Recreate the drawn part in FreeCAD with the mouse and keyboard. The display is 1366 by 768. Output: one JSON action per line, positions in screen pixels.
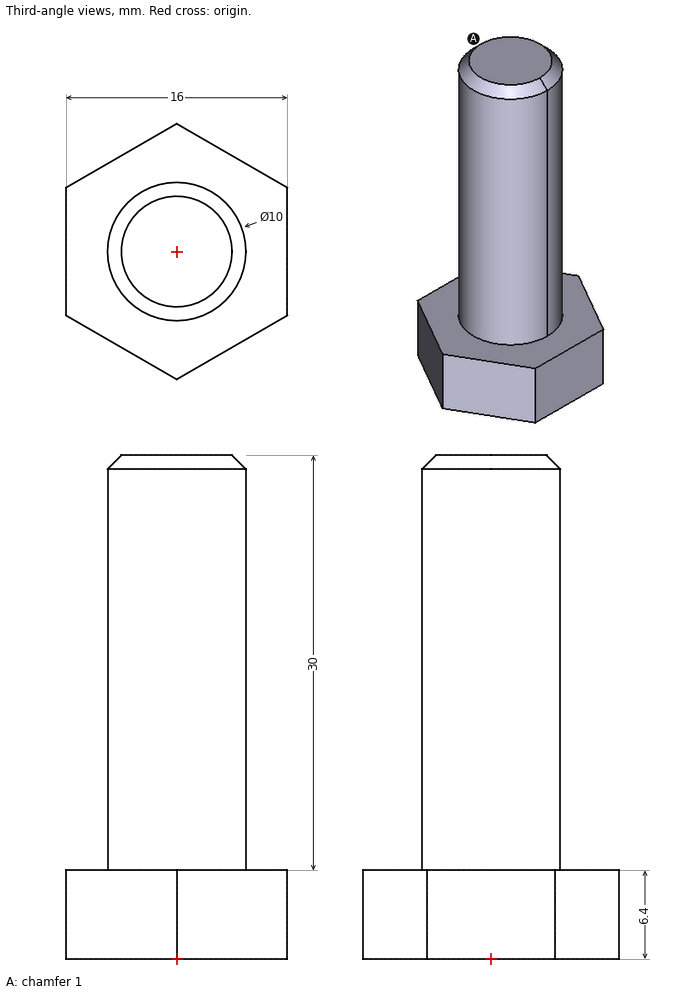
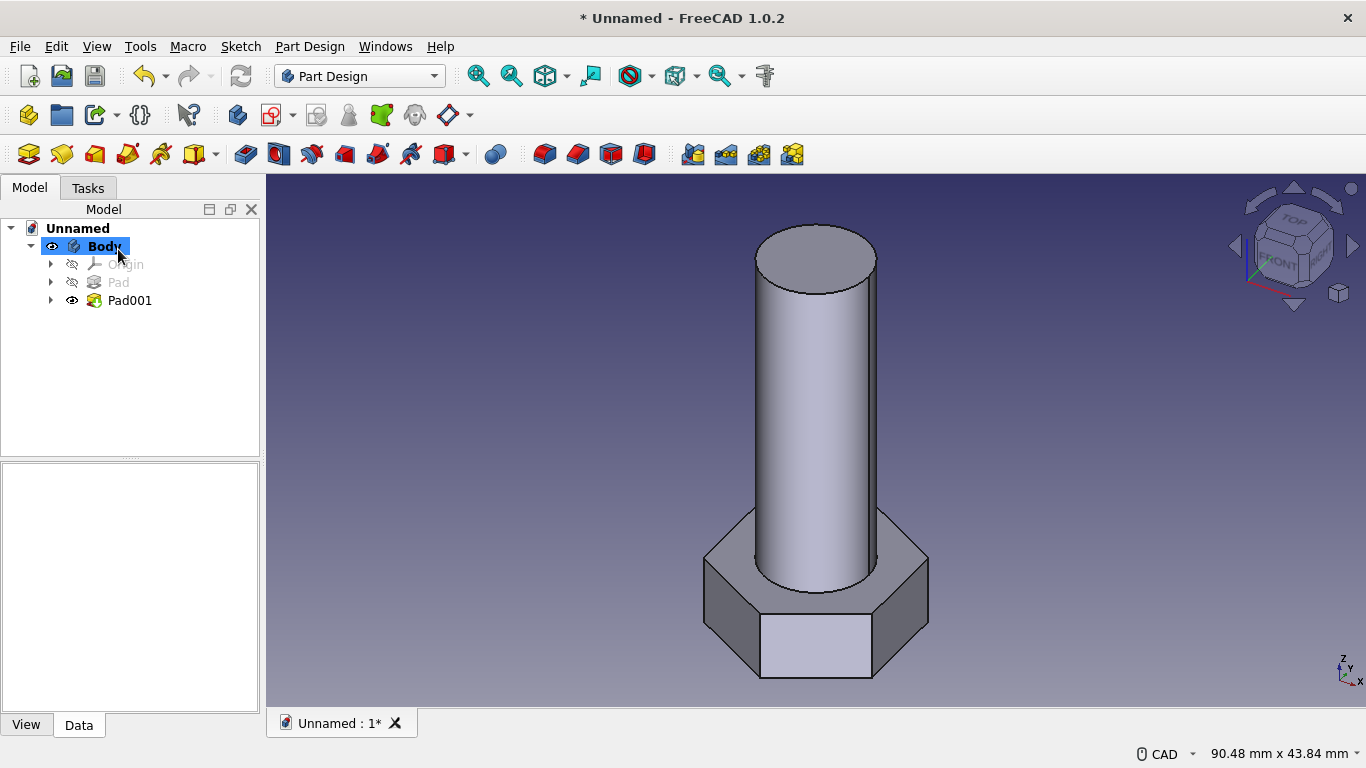
{"action": "left_click", "coordinate": [756, 262]}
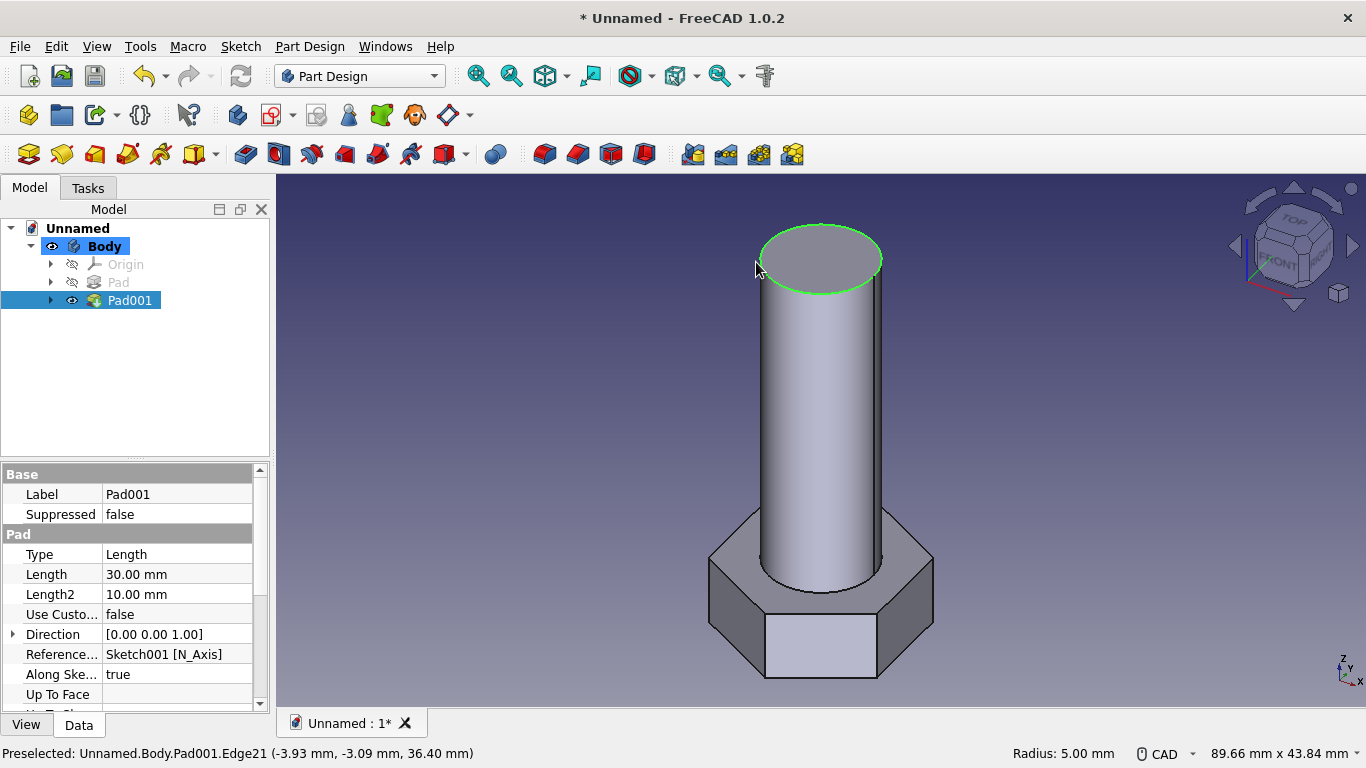
{"action": "left_click", "coordinate": [578, 154]}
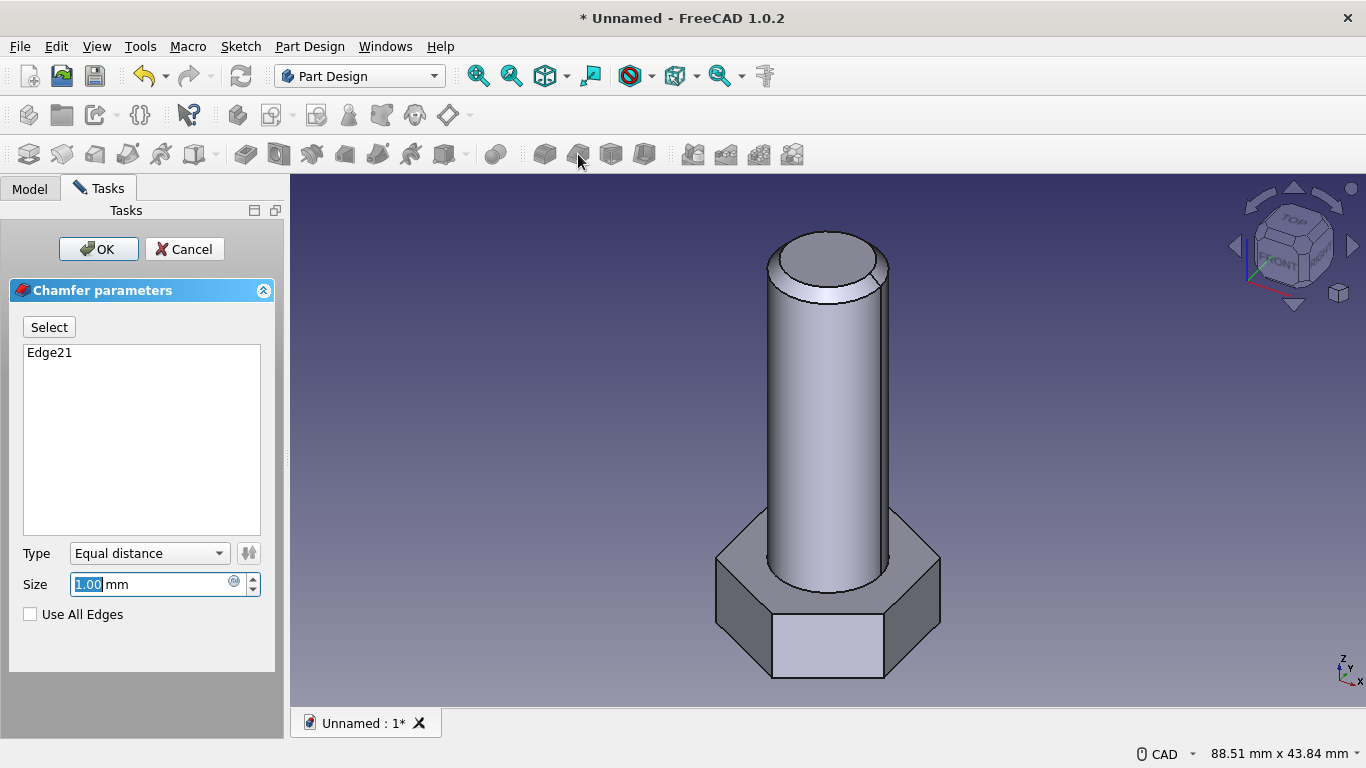
{"action": "type", "text": "1"}
{"action": "key", "text": "Tab"}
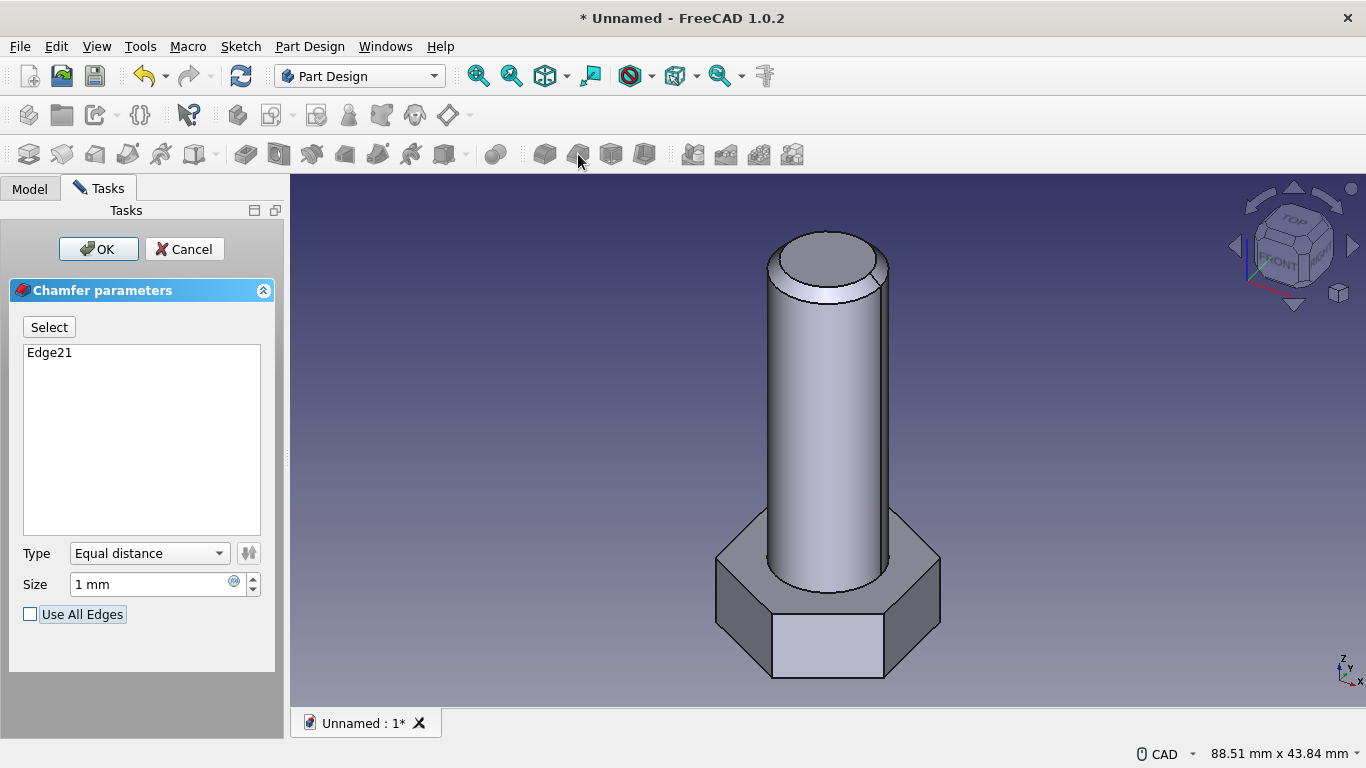
{"action": "left_click", "coordinate": [99, 249]}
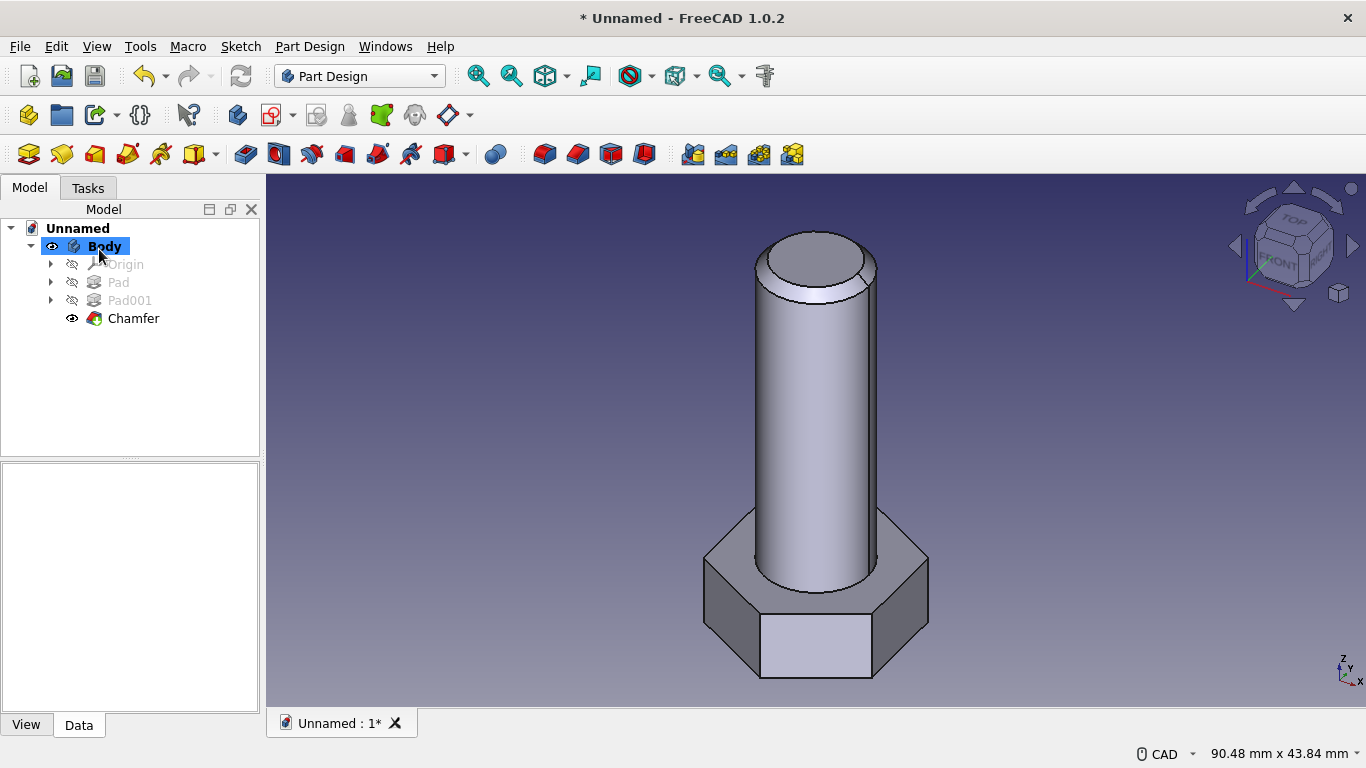
{"action": "key", "text": "0"}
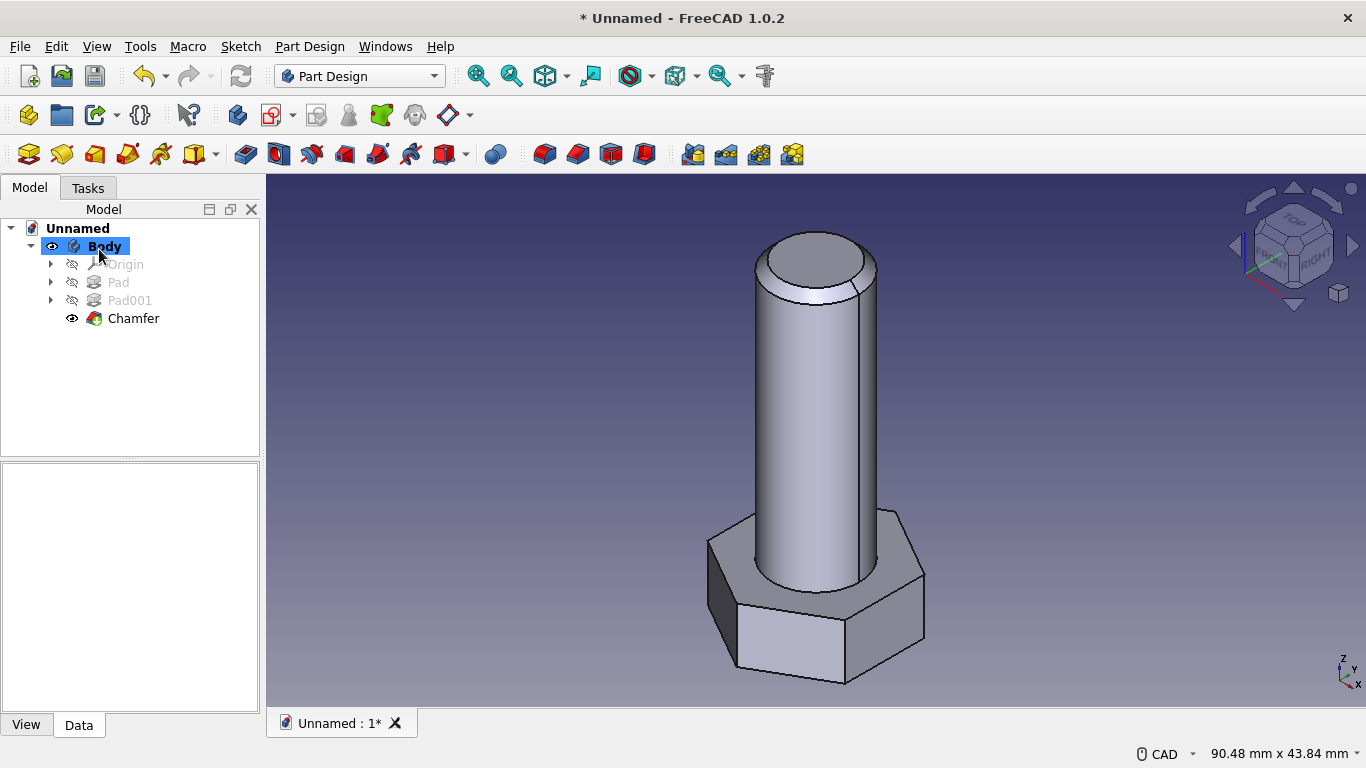
{"action": "key", "text": "v f"}